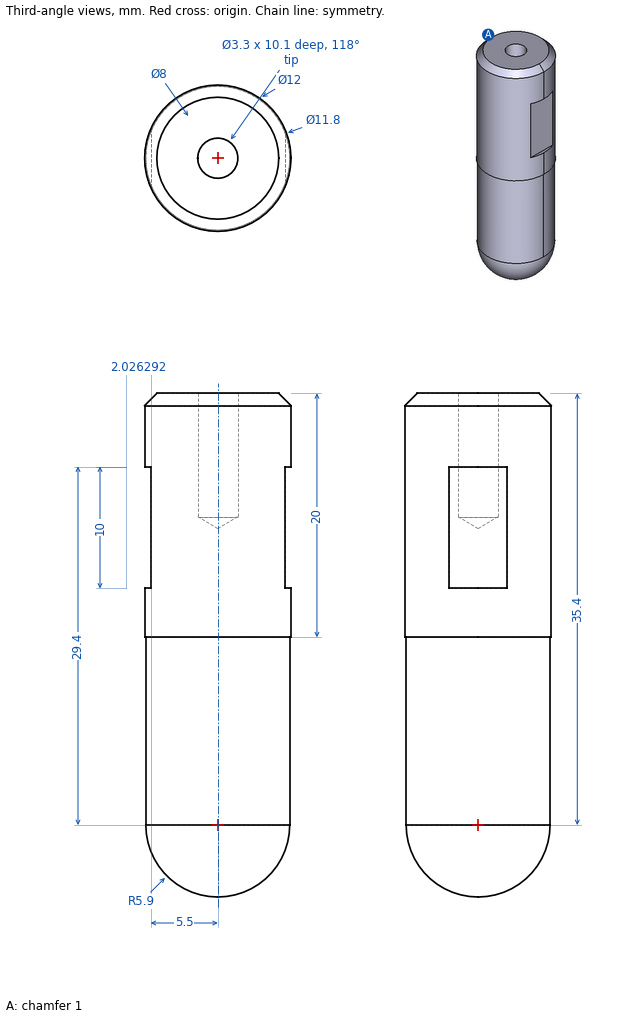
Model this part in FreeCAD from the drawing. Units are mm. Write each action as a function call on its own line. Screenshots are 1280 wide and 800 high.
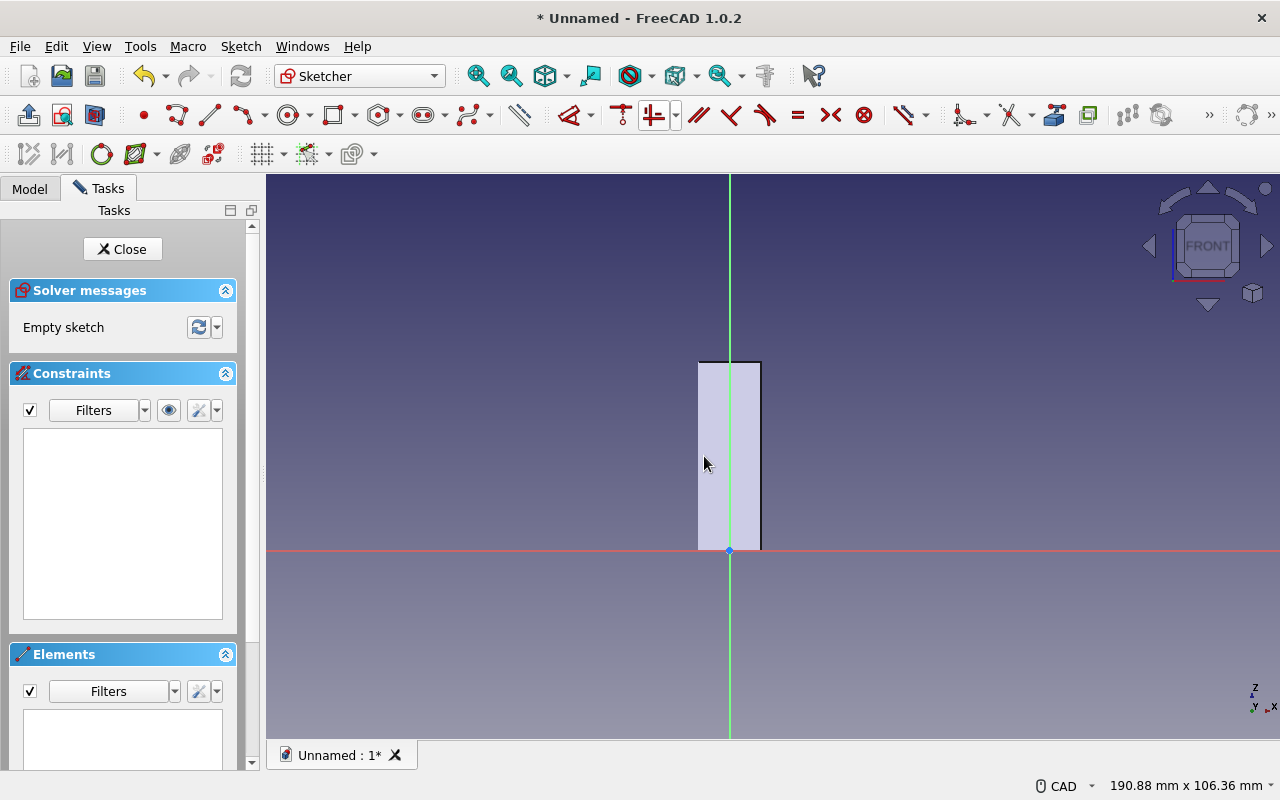
scroll(715, 577, up, 12)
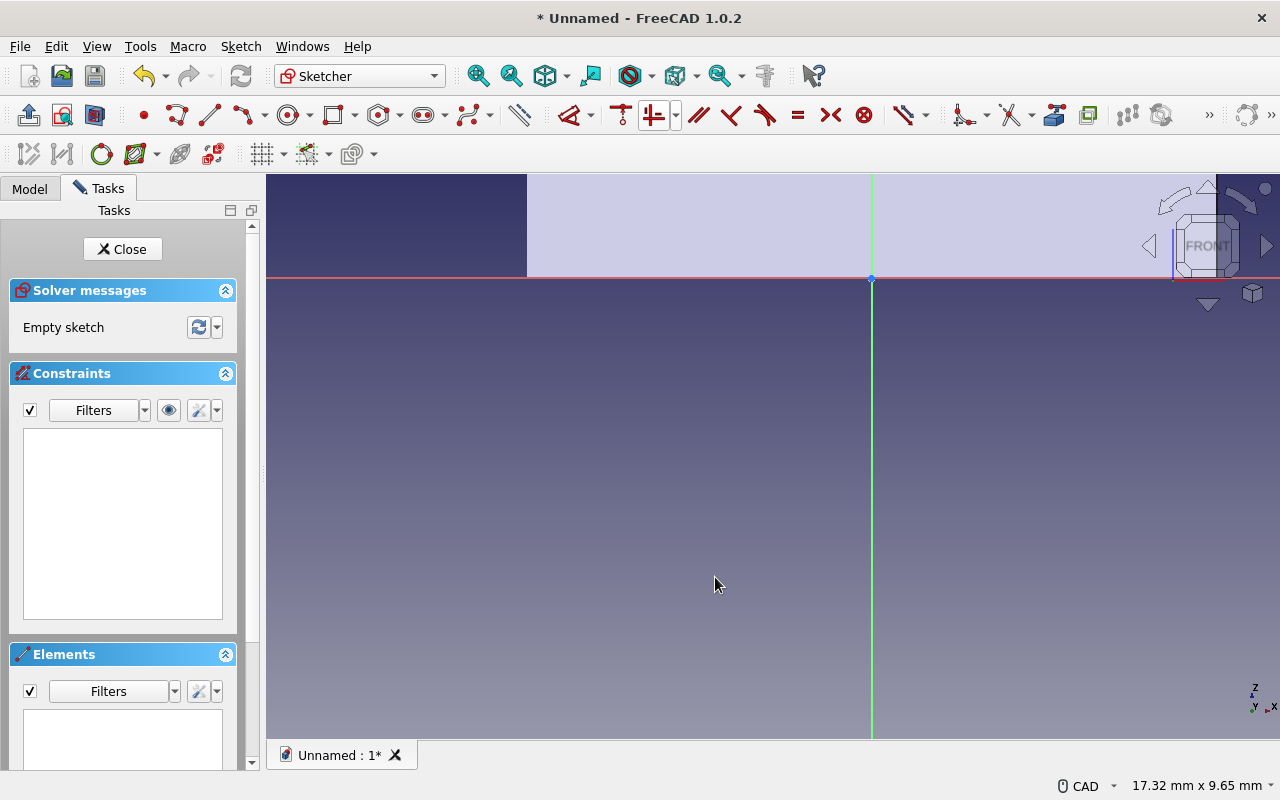
click(177, 116)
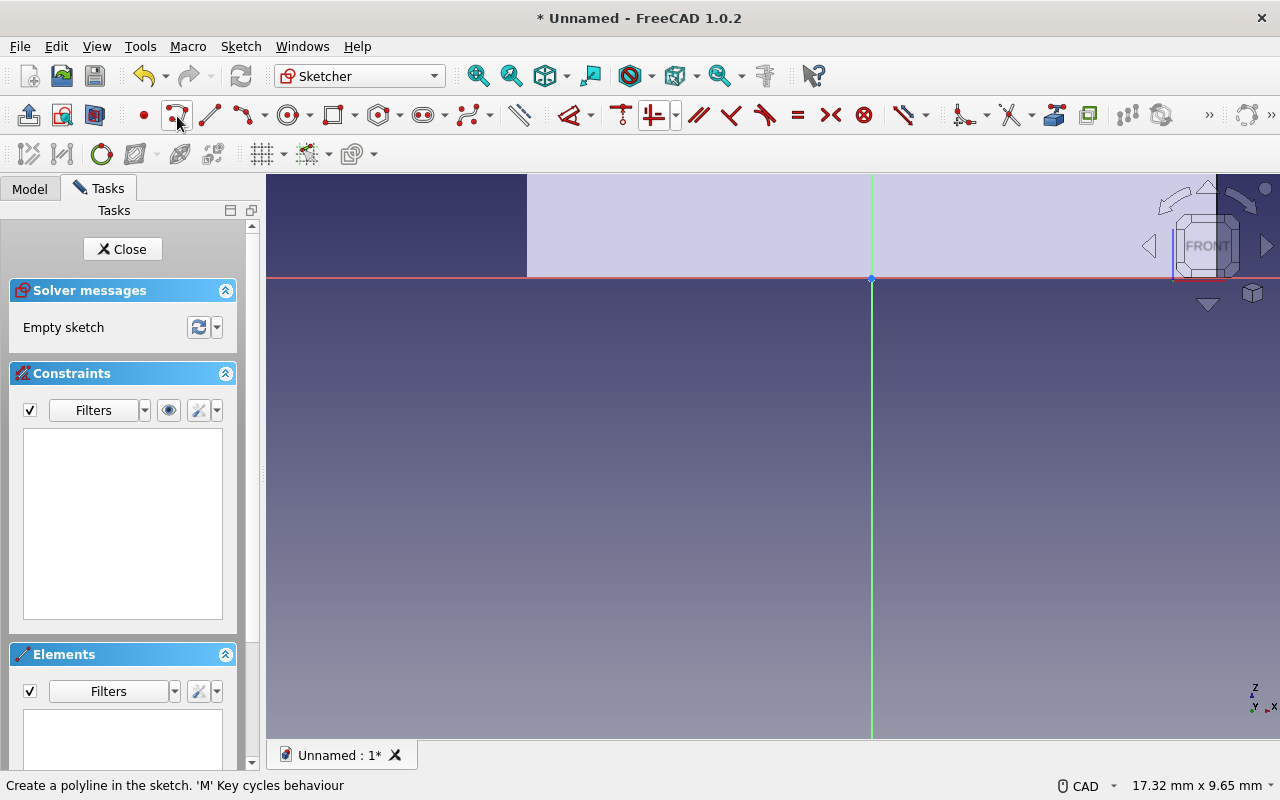
click(526, 278)
click(872, 278)
click(863, 623)
right_click(863, 623)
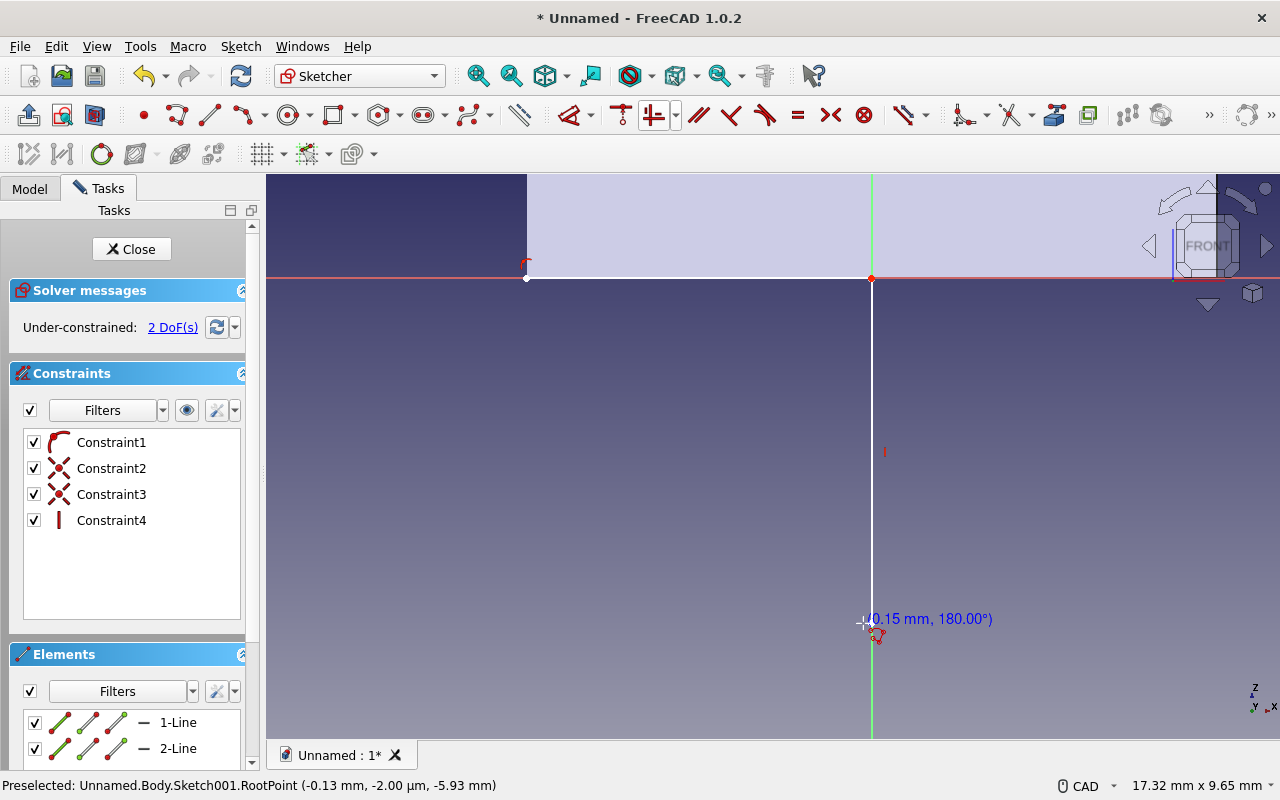
click(242, 116)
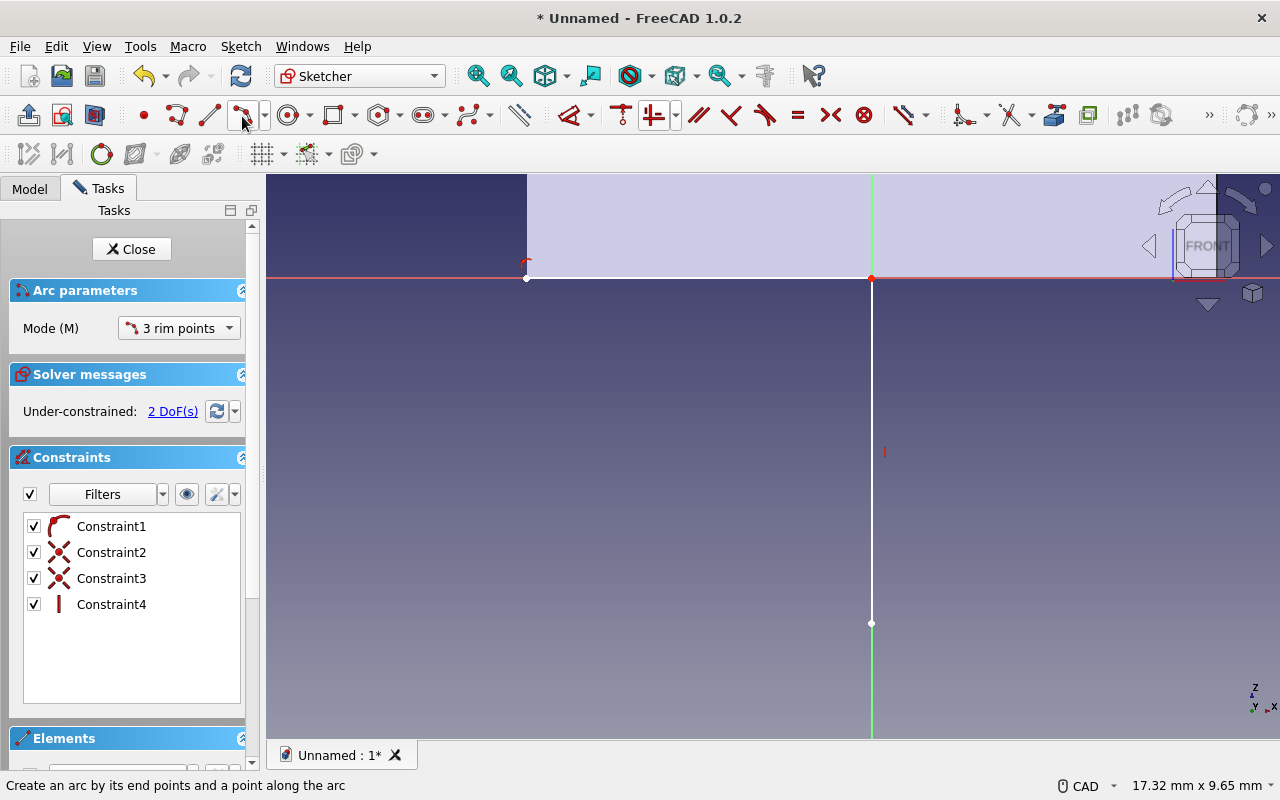
click(872, 624)
click(526, 278)
click(627, 522)
key(Escape)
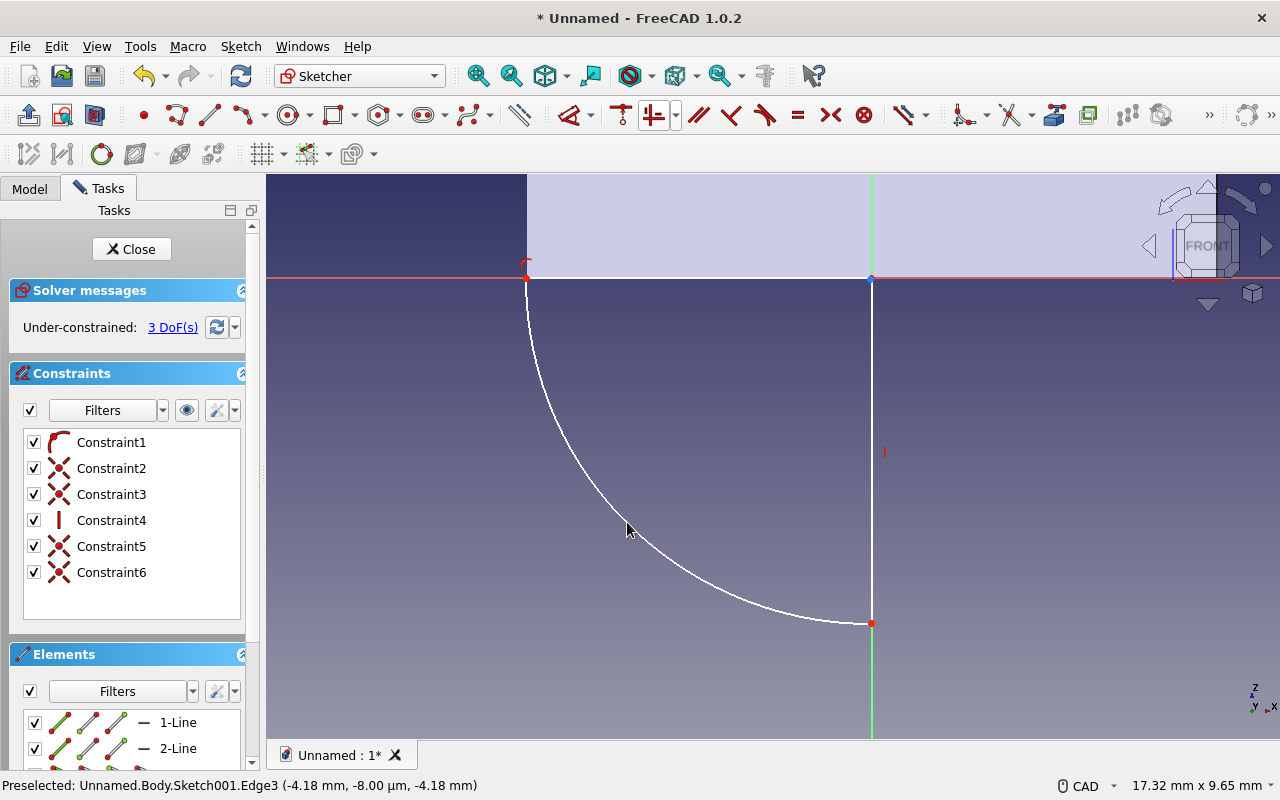
scroll(871, 279, up, 21)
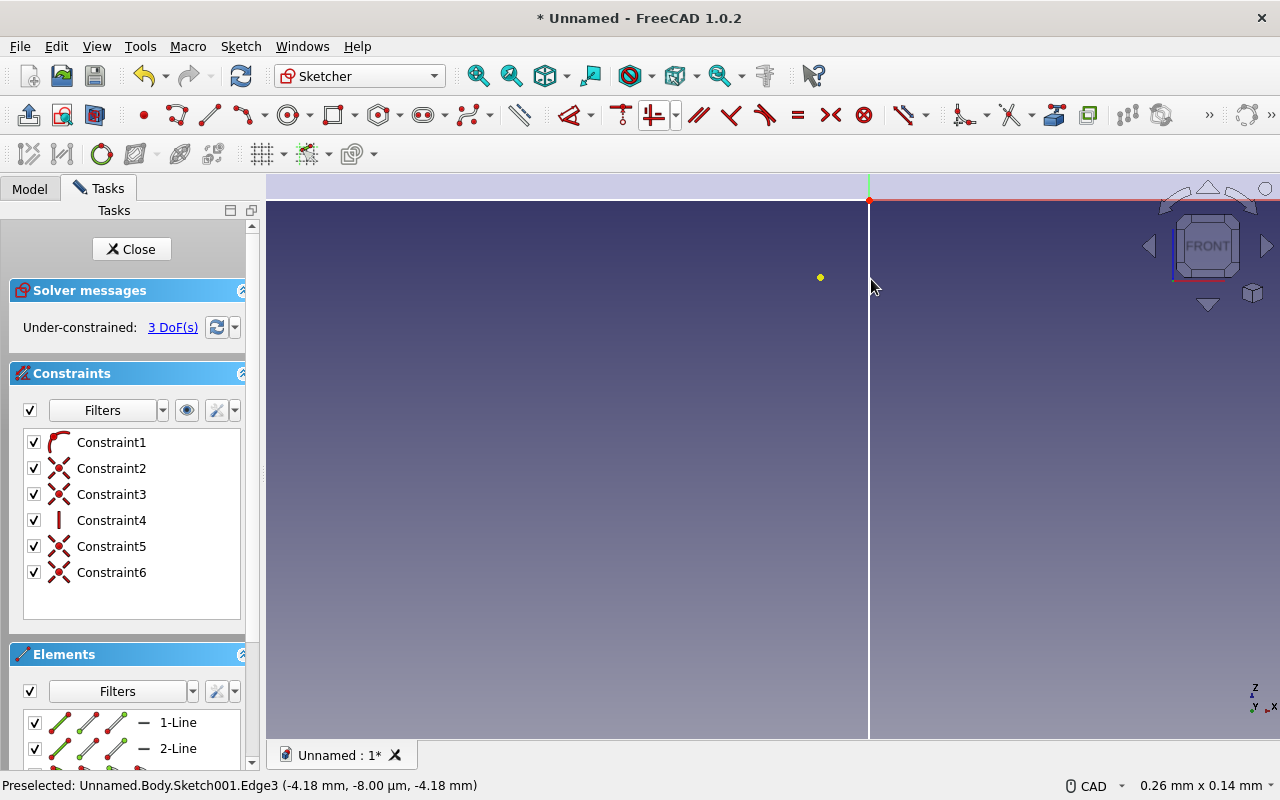
drag(811, 190, 879, 287)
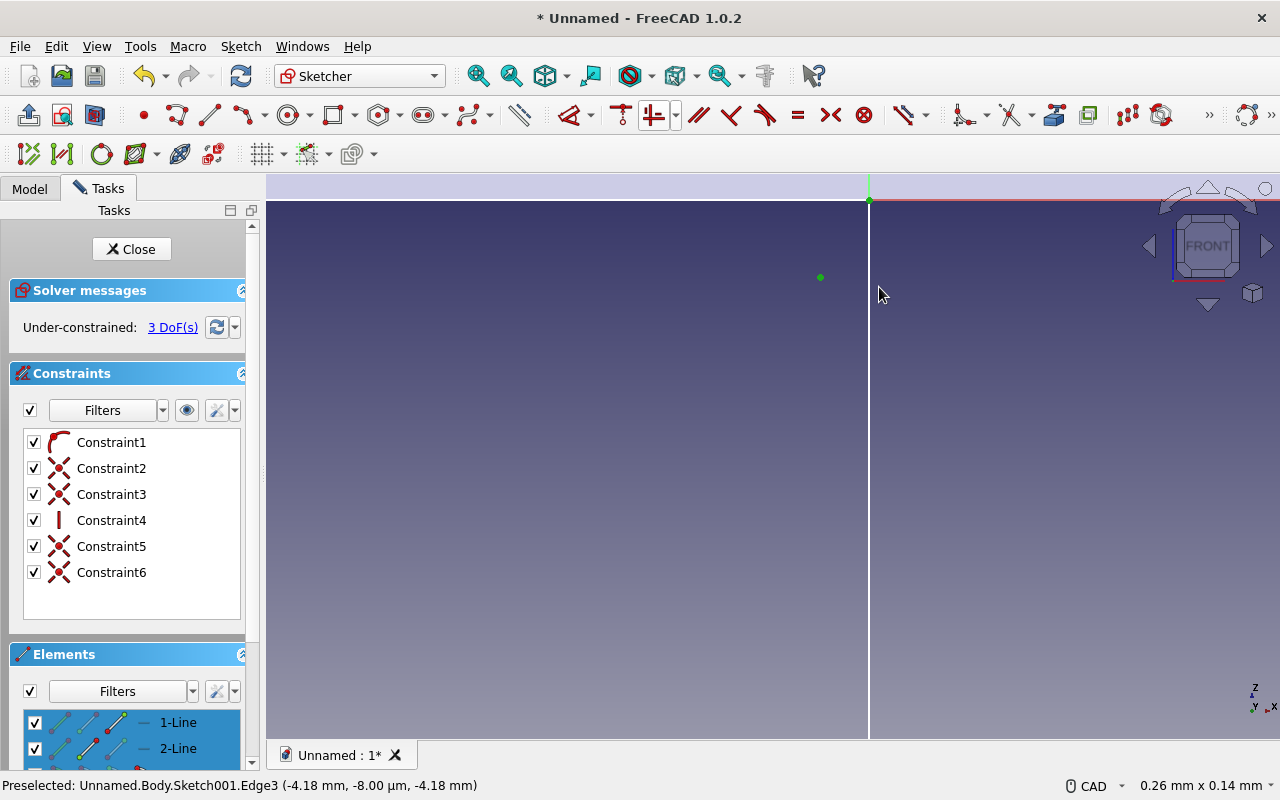
click(621, 116)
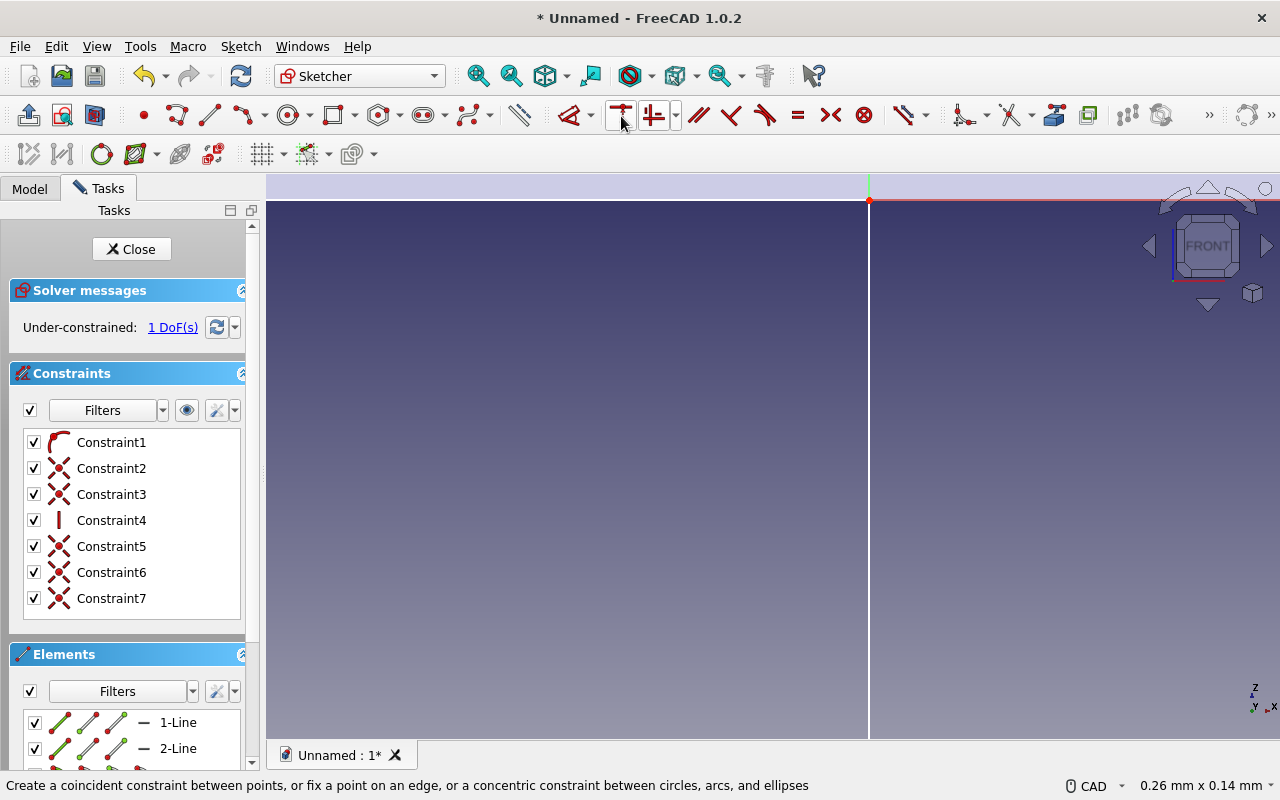
click(568, 116)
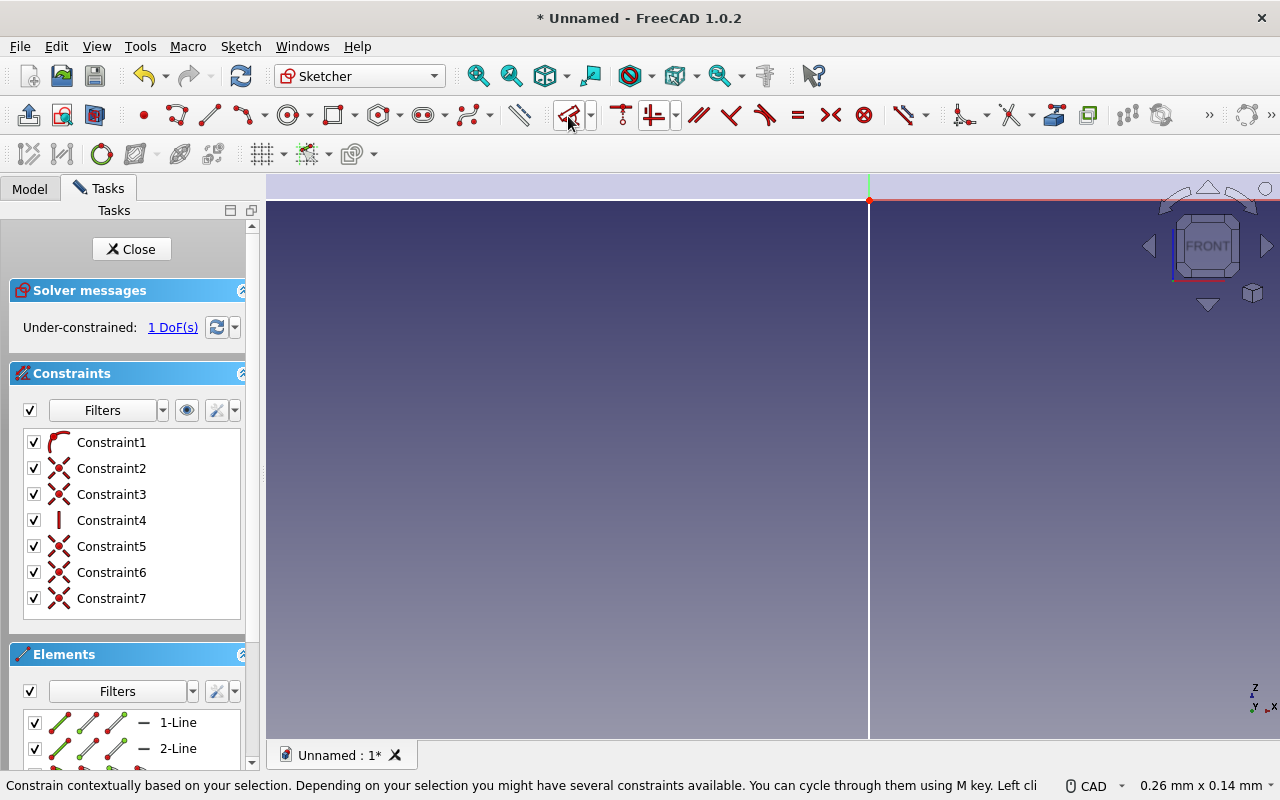
scroll(704, 456, down, 15)